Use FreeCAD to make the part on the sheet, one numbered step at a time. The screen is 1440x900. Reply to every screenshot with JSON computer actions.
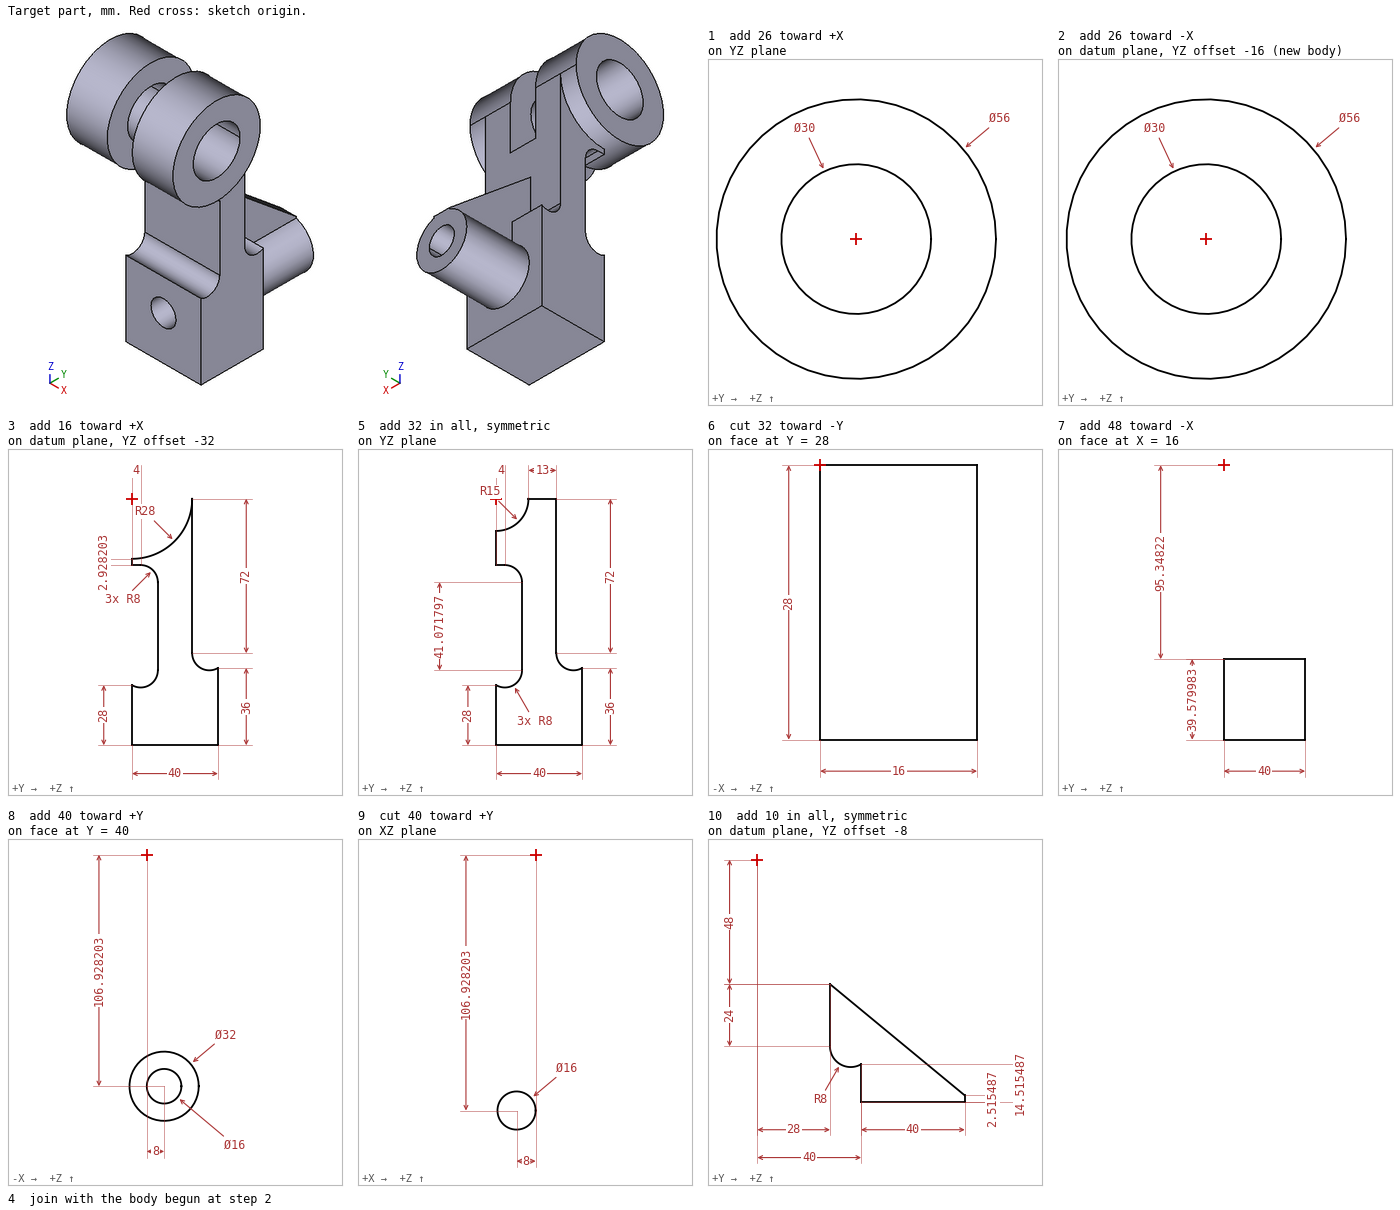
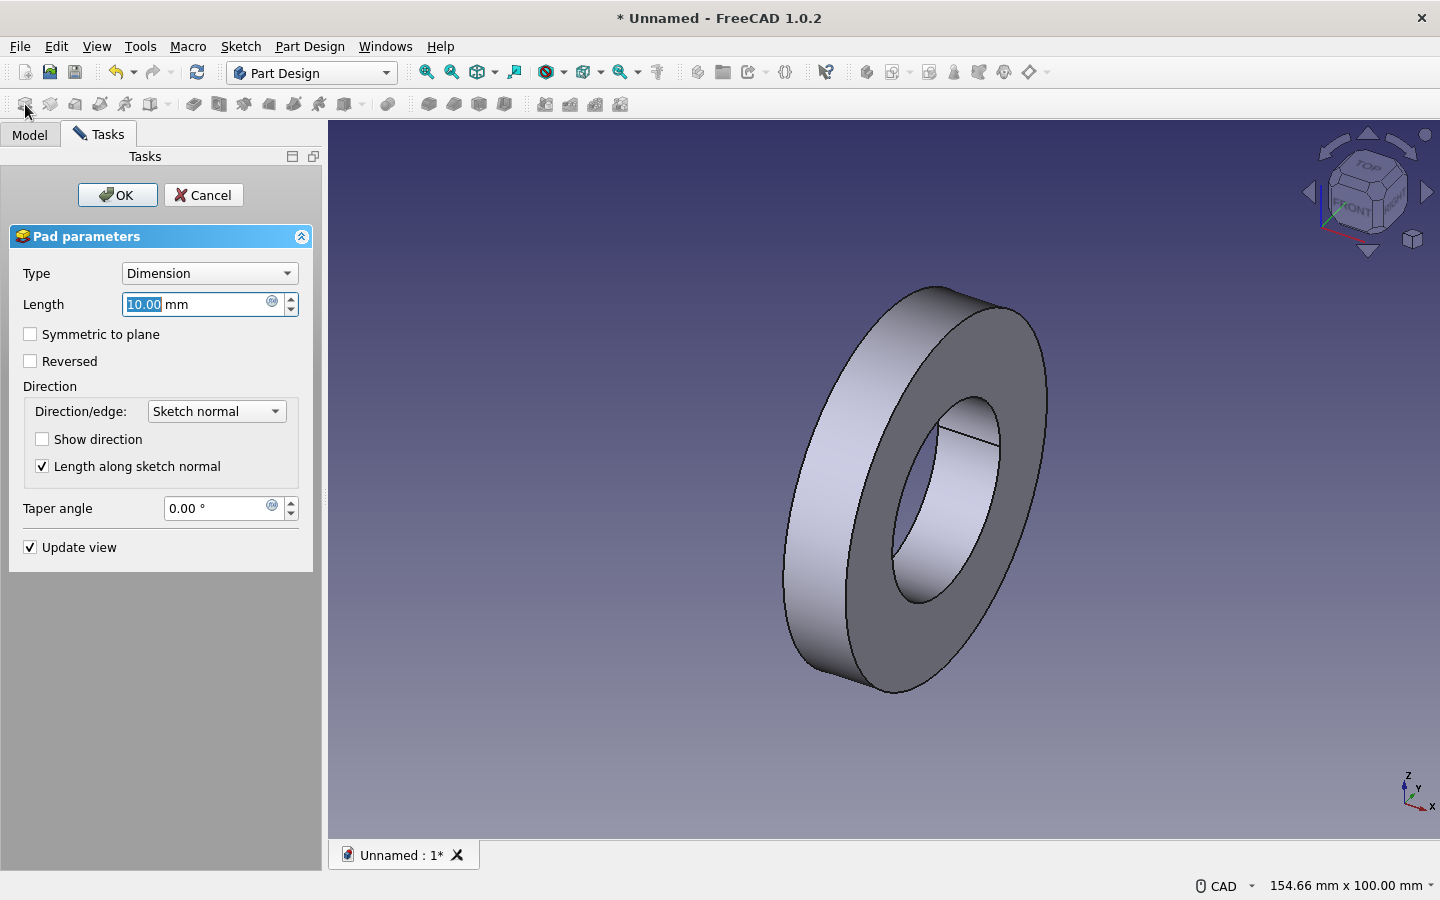
{"action": "type", "text": "26"}
{"action": "key", "text": "Tab"}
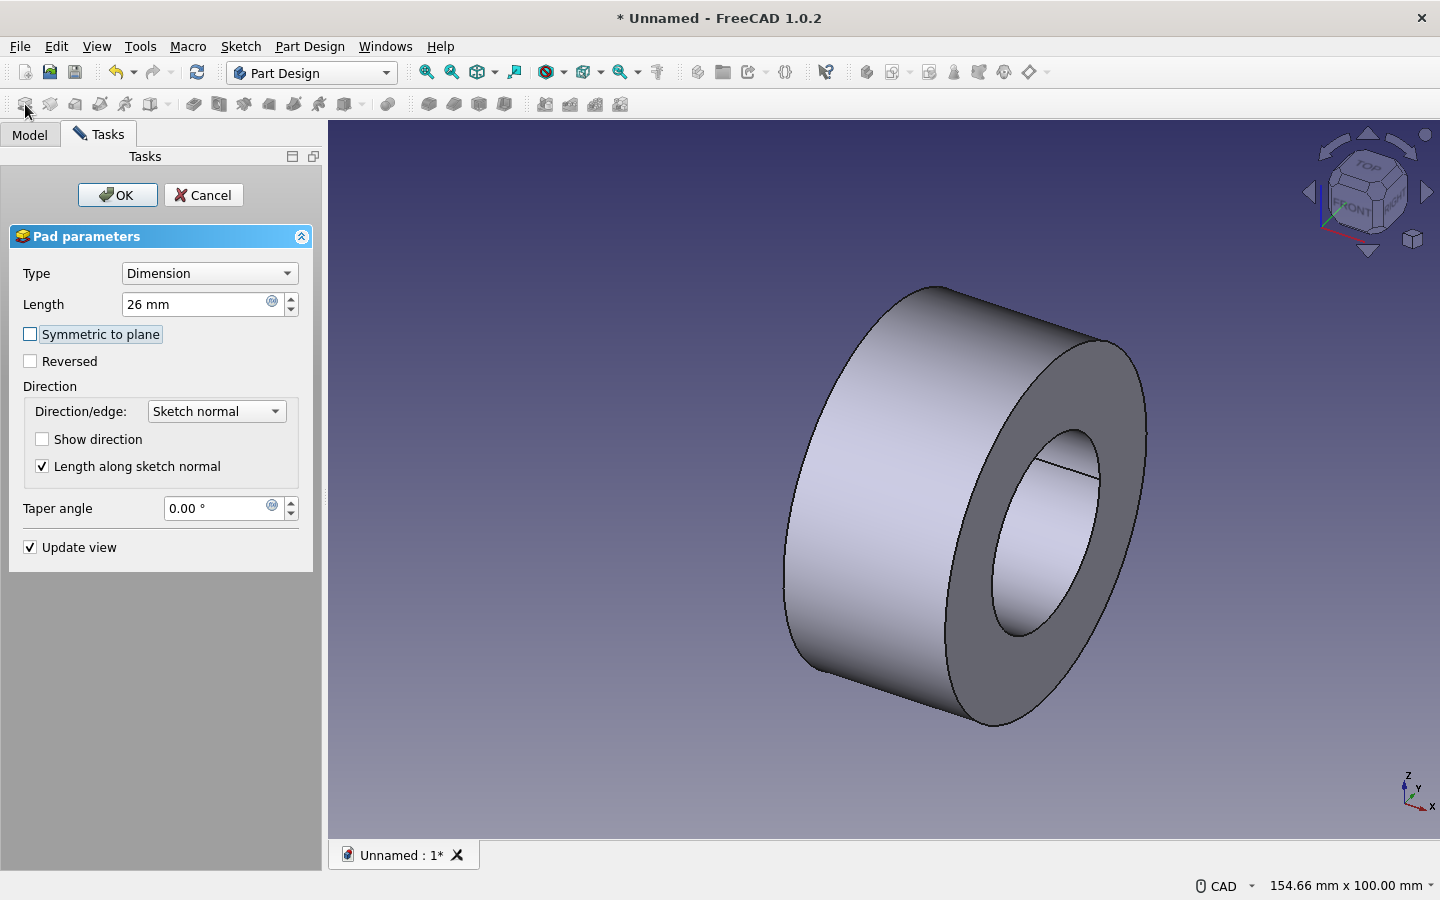
{"action": "left_click", "coordinate": [118, 195]}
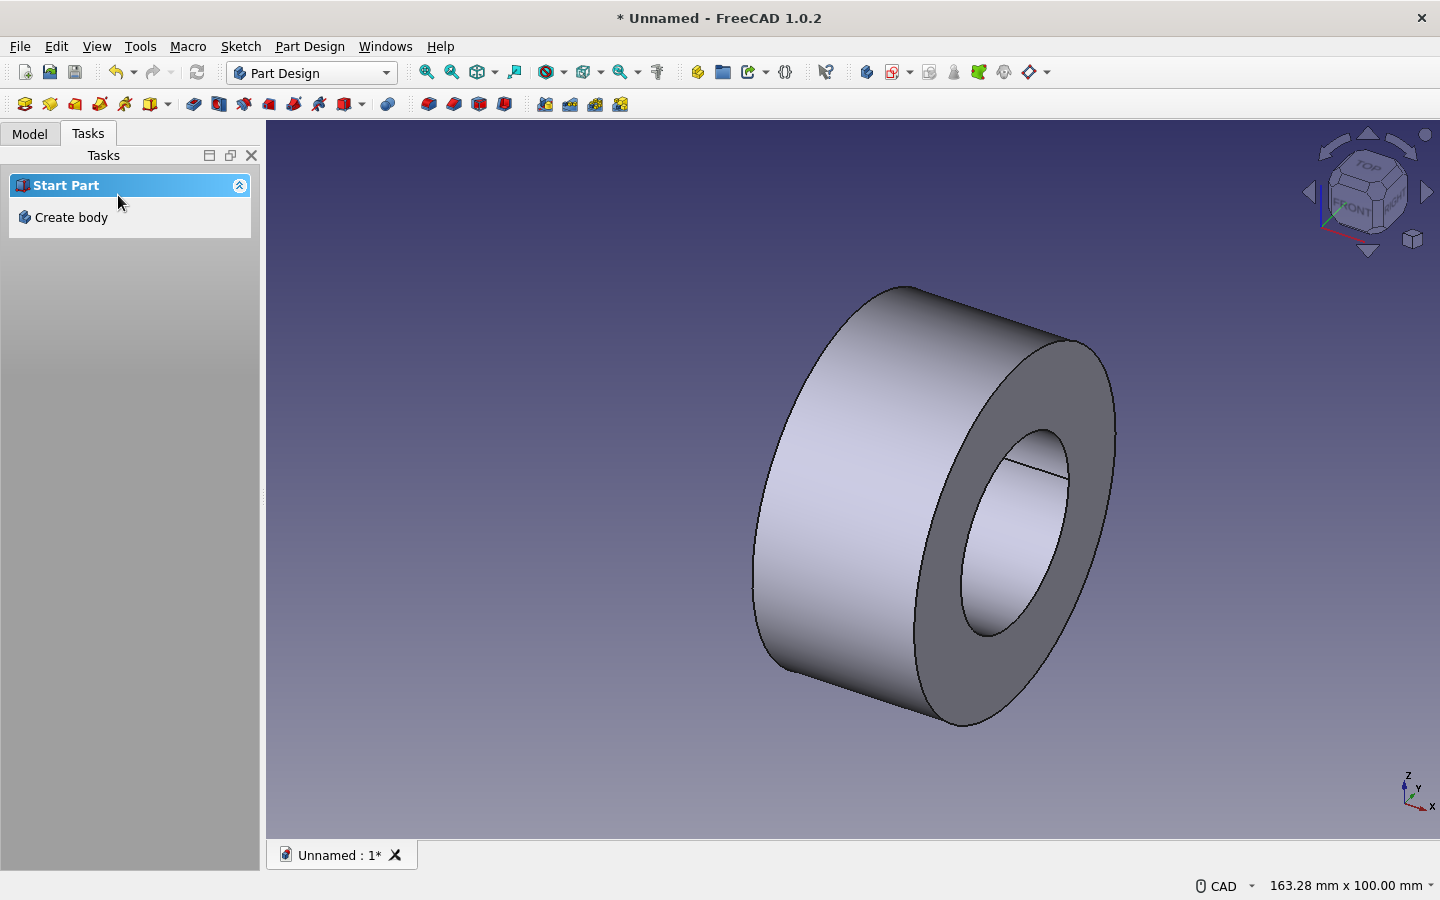
{"action": "left_click", "coordinate": [867, 72]}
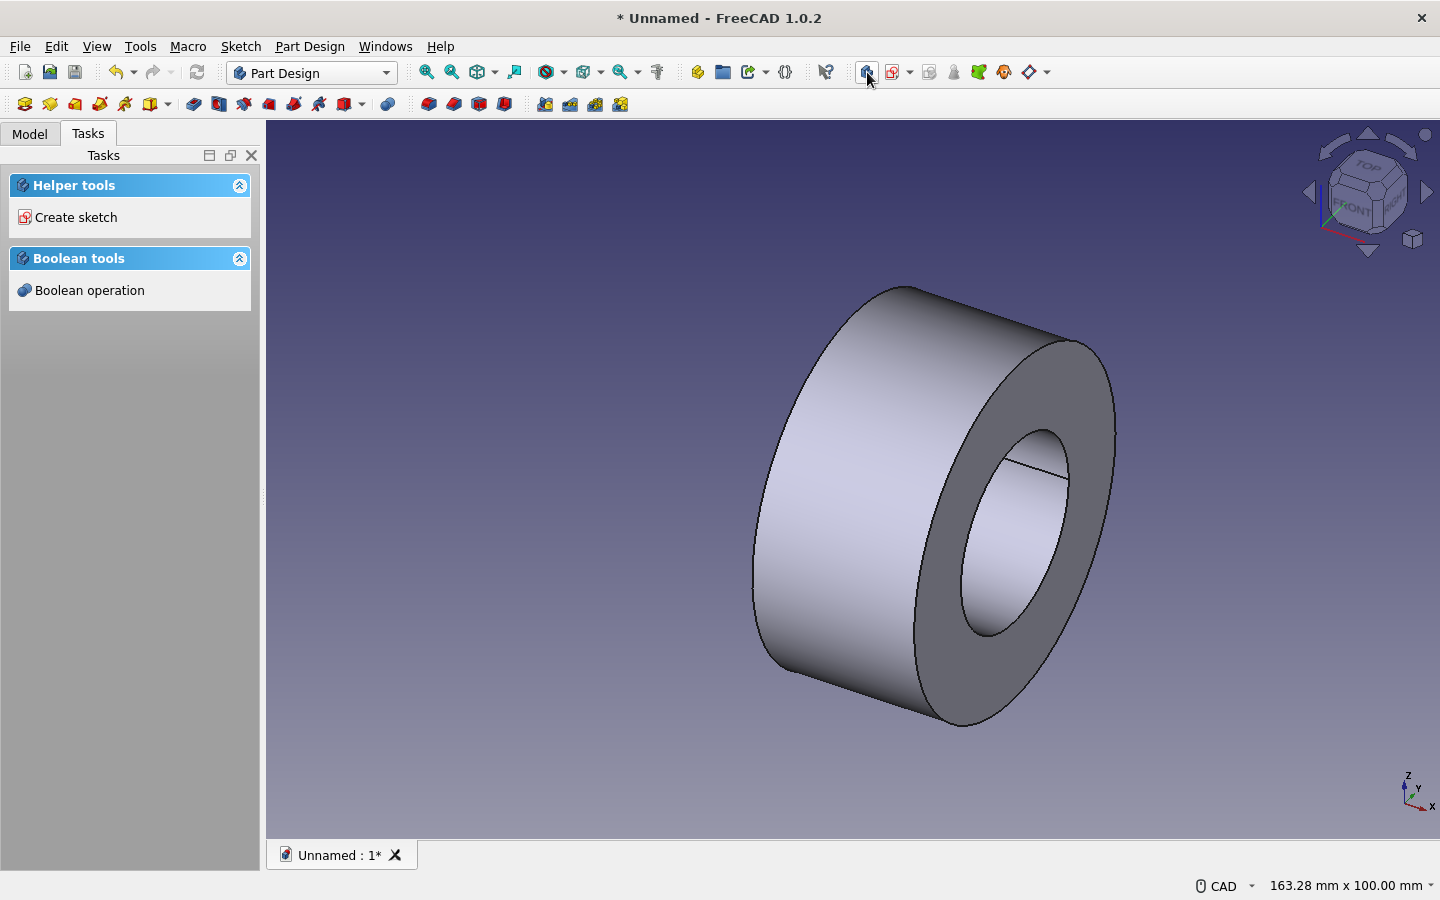
{"action": "left_click", "coordinate": [30, 134]}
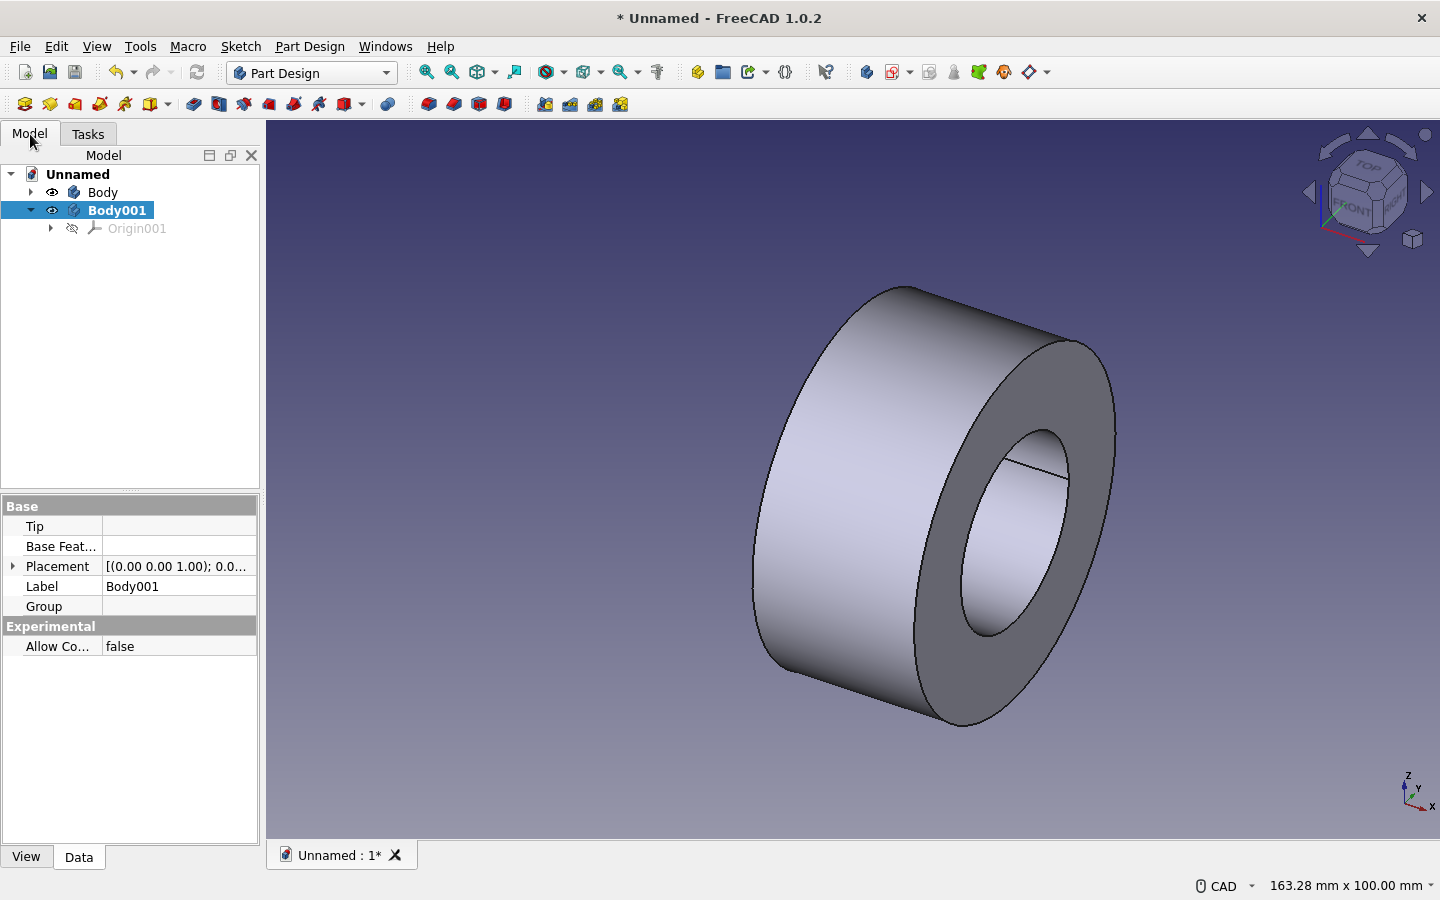
{"action": "left_click", "coordinate": [51, 228]}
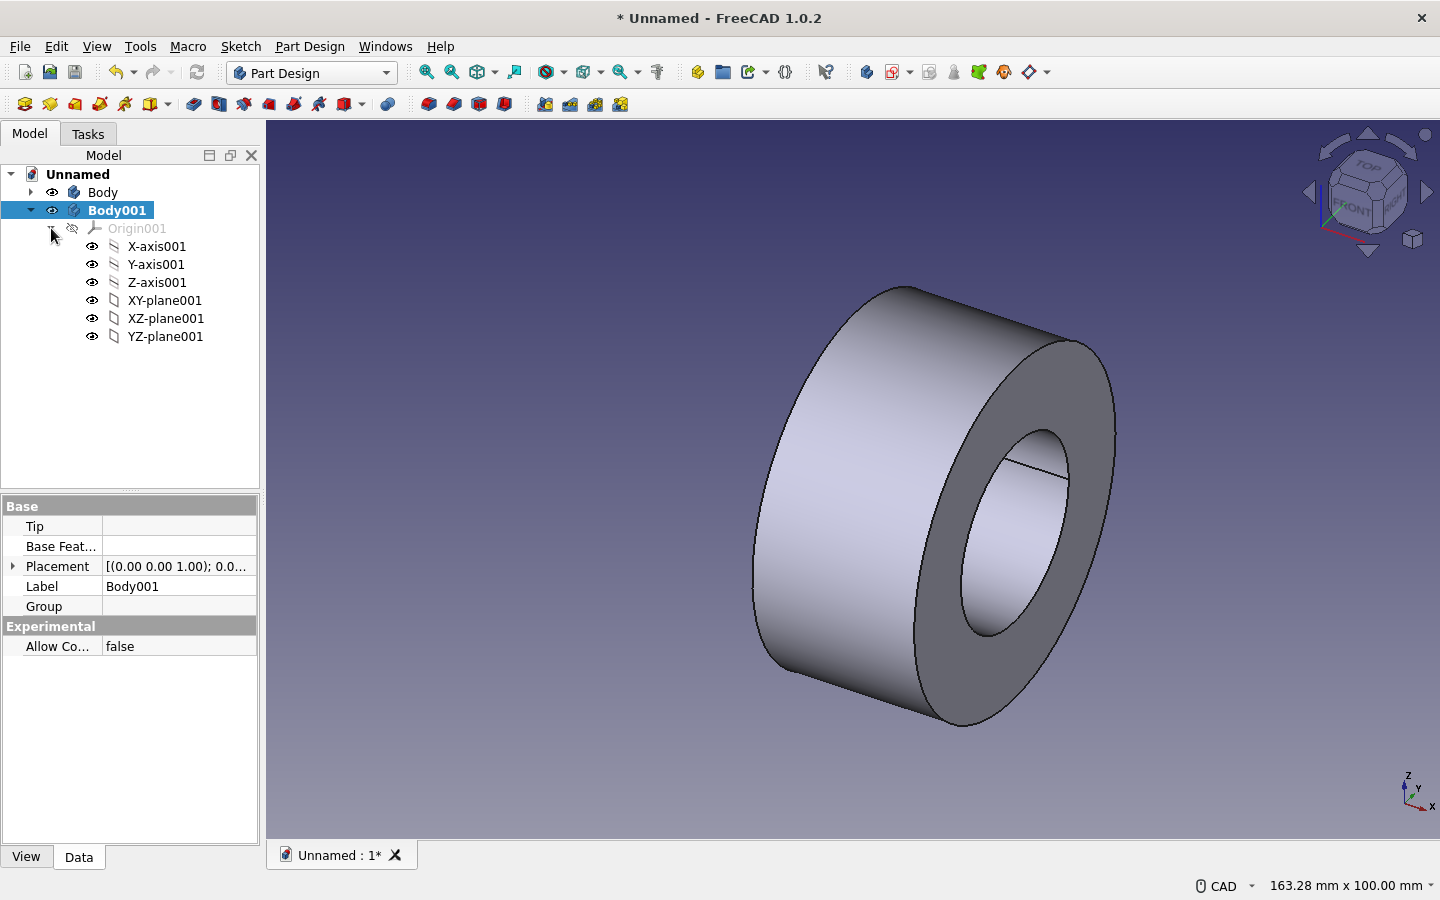
{"action": "left_click", "coordinate": [137, 336]}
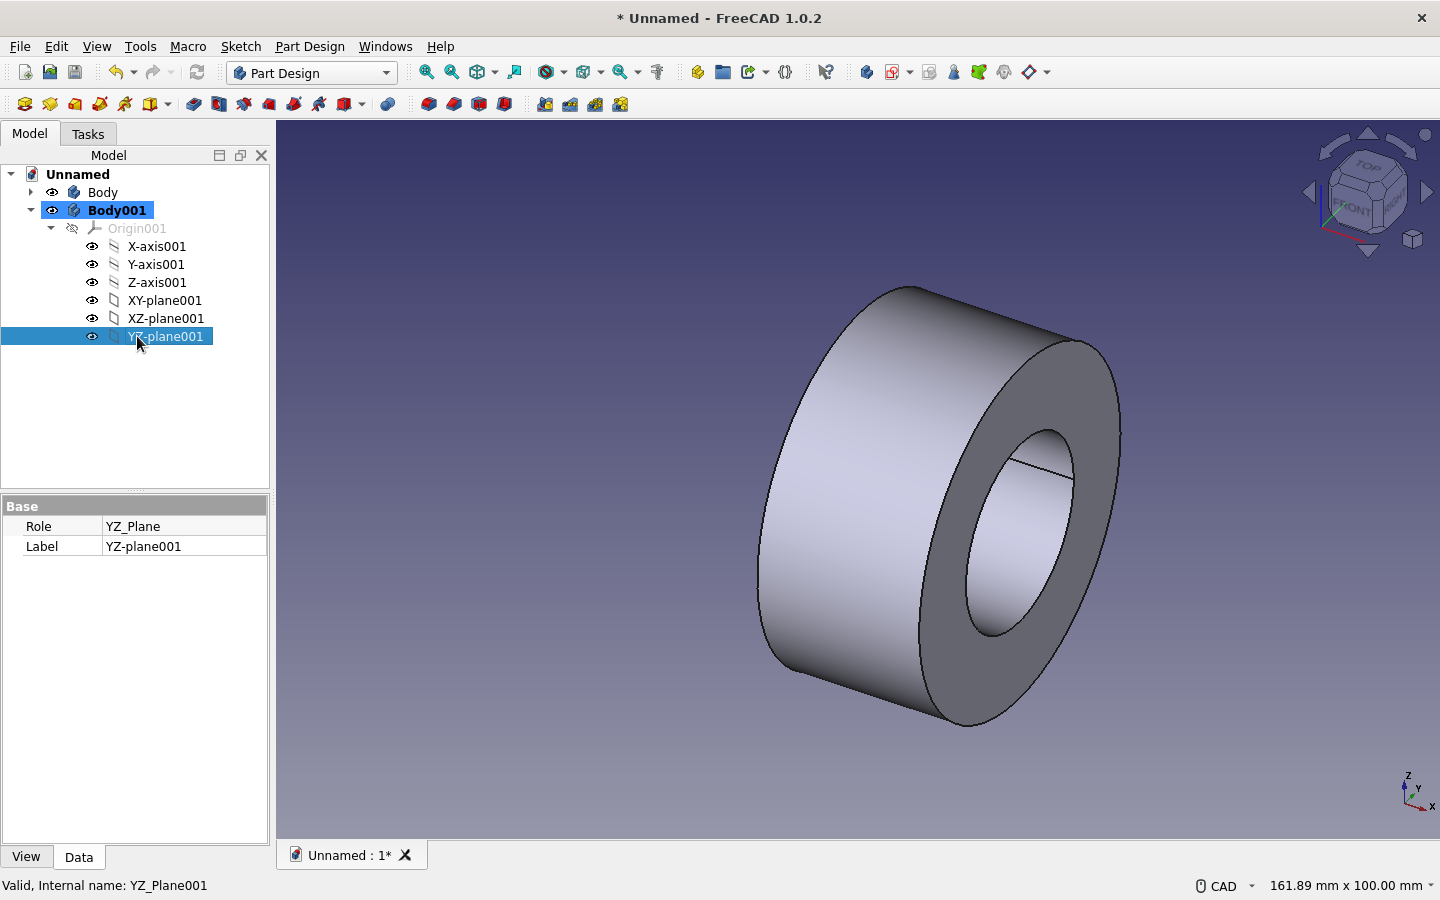
{"action": "left_click", "coordinate": [1028, 72]}